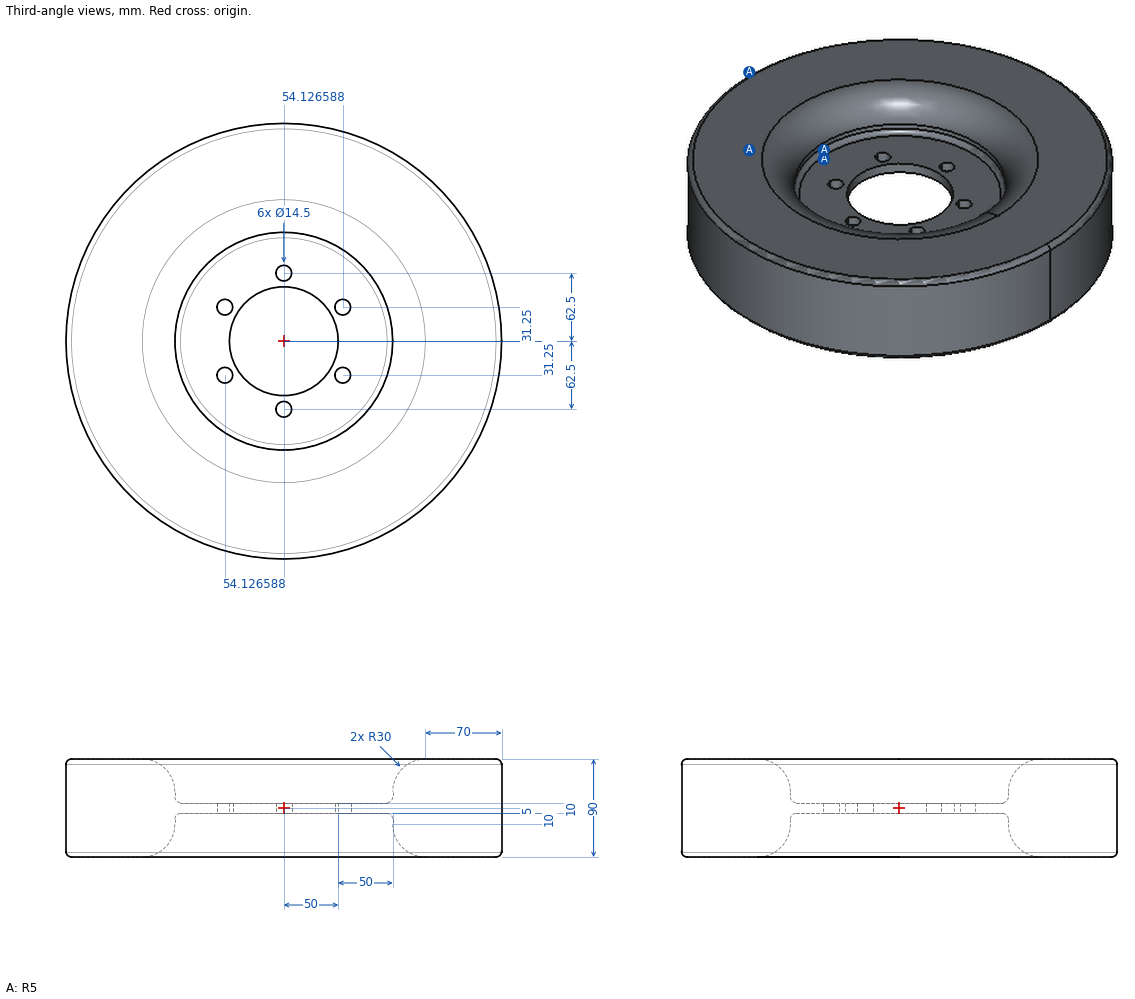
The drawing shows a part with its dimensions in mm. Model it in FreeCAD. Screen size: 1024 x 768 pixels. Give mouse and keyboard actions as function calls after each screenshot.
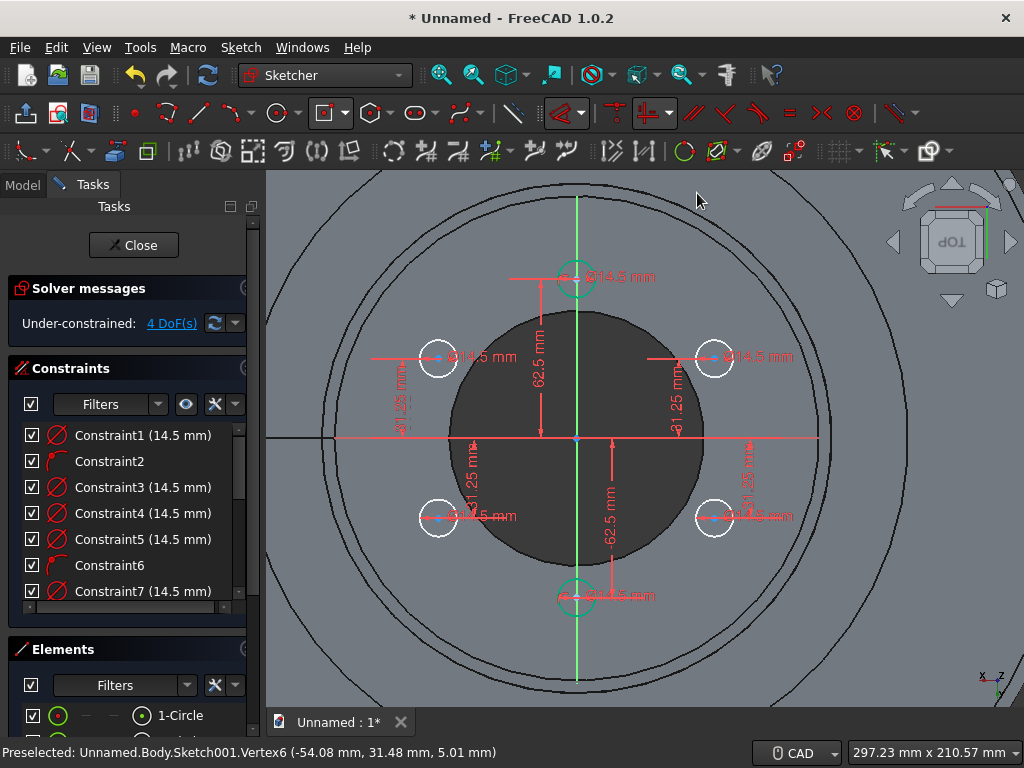
click(438, 518)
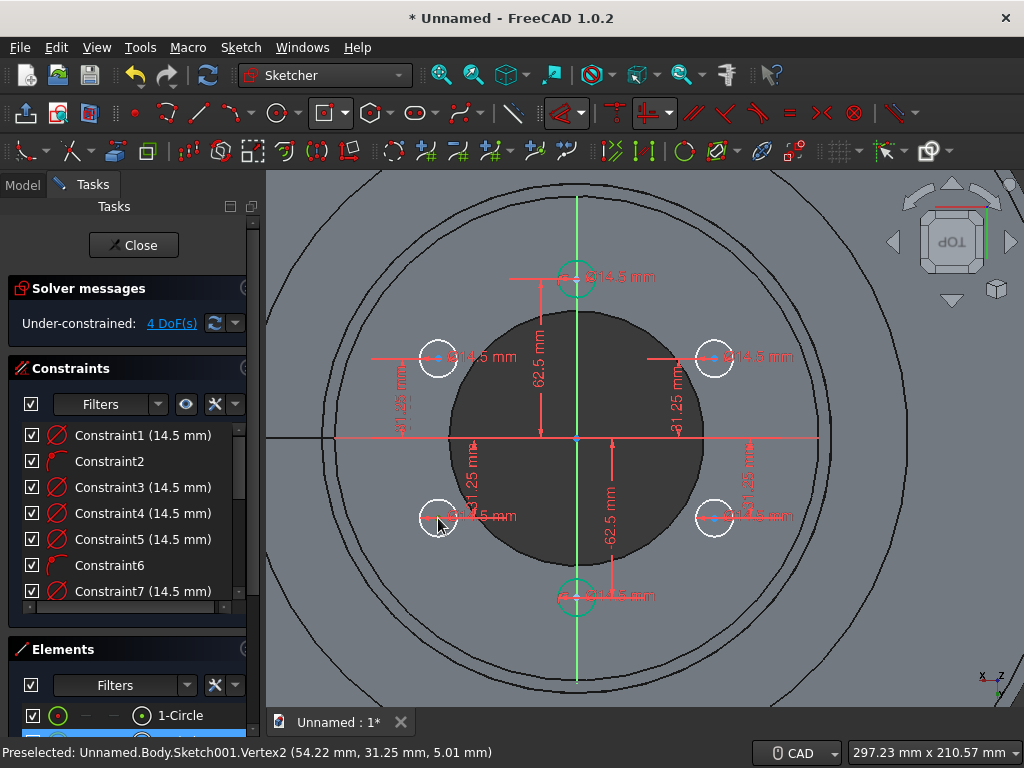
click(584, 114)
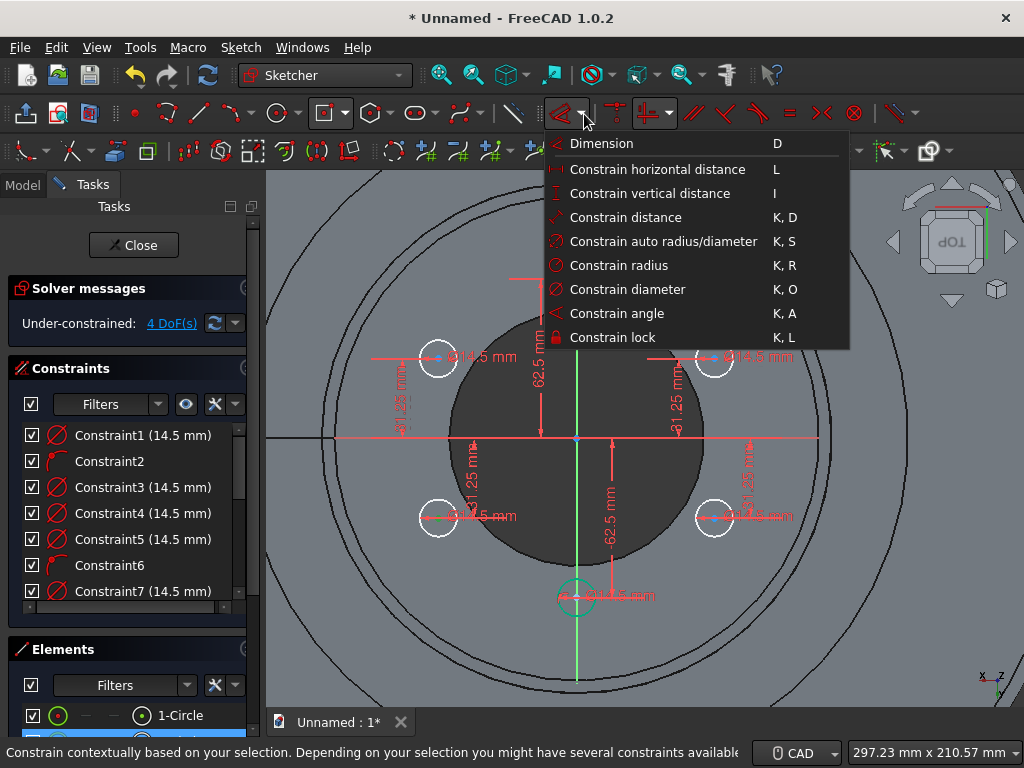
click(697, 169)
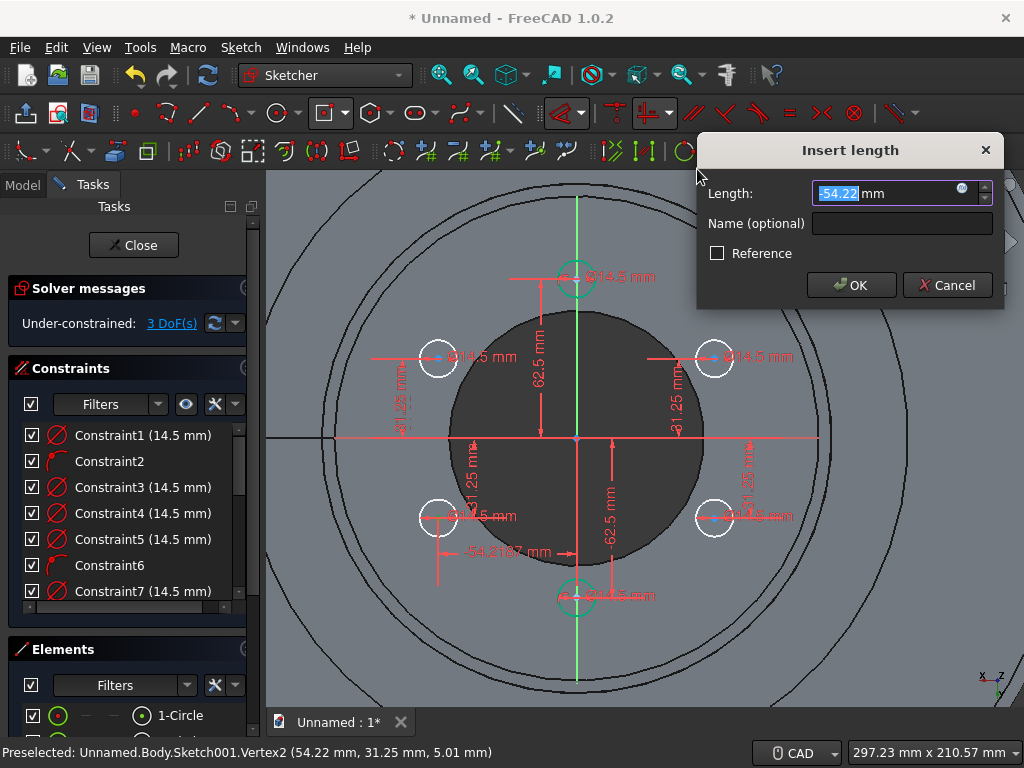
text(-54.126588)
key(Return)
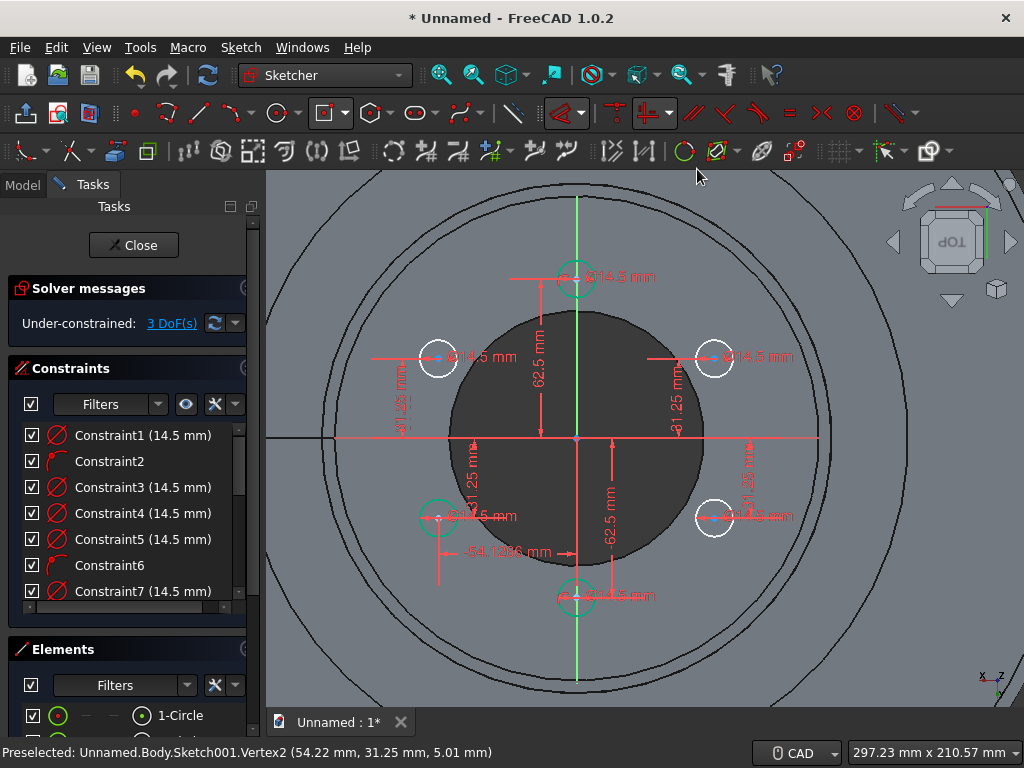
click(438, 359)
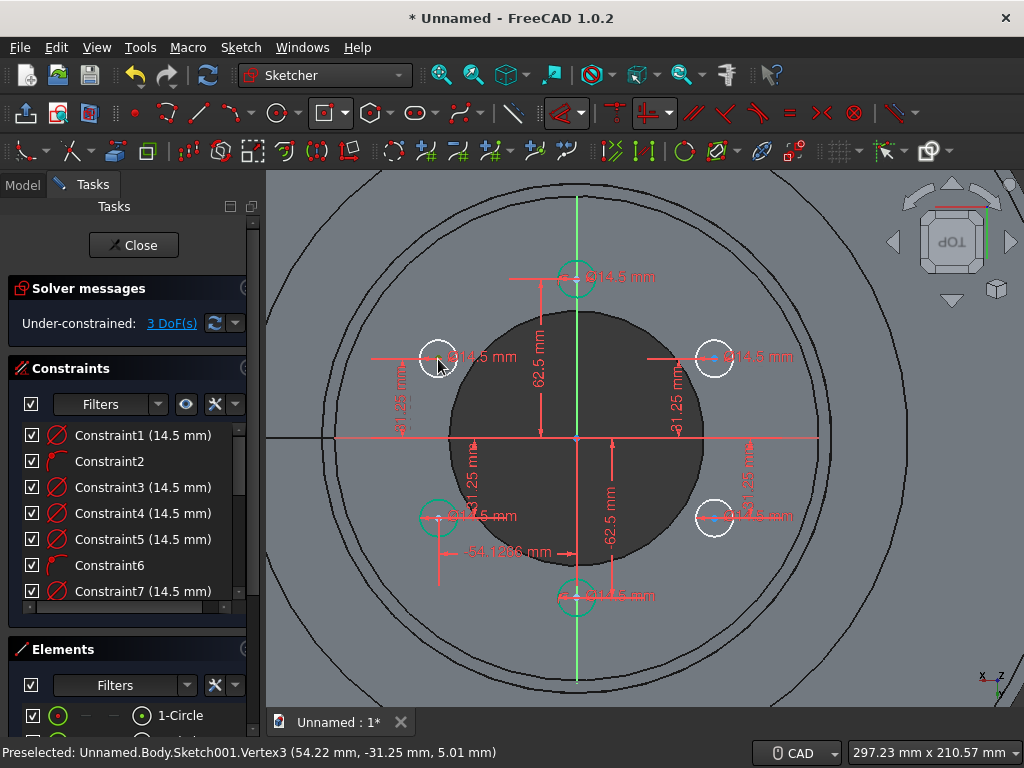
key(l)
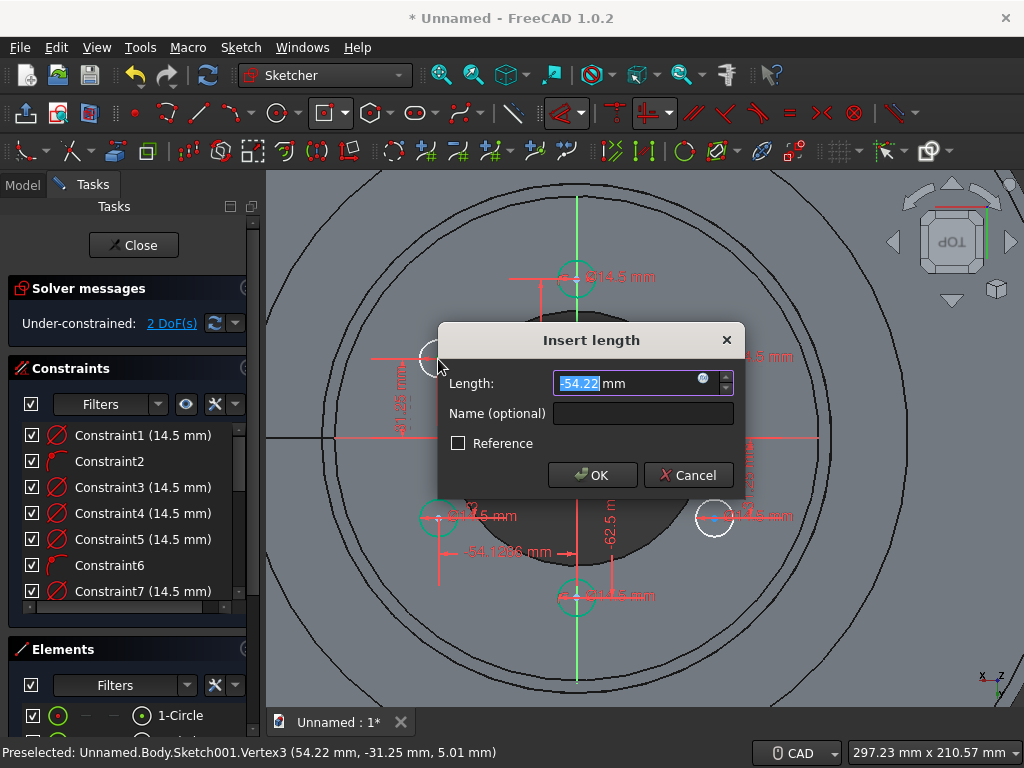
text(-54.126588)
key(Return)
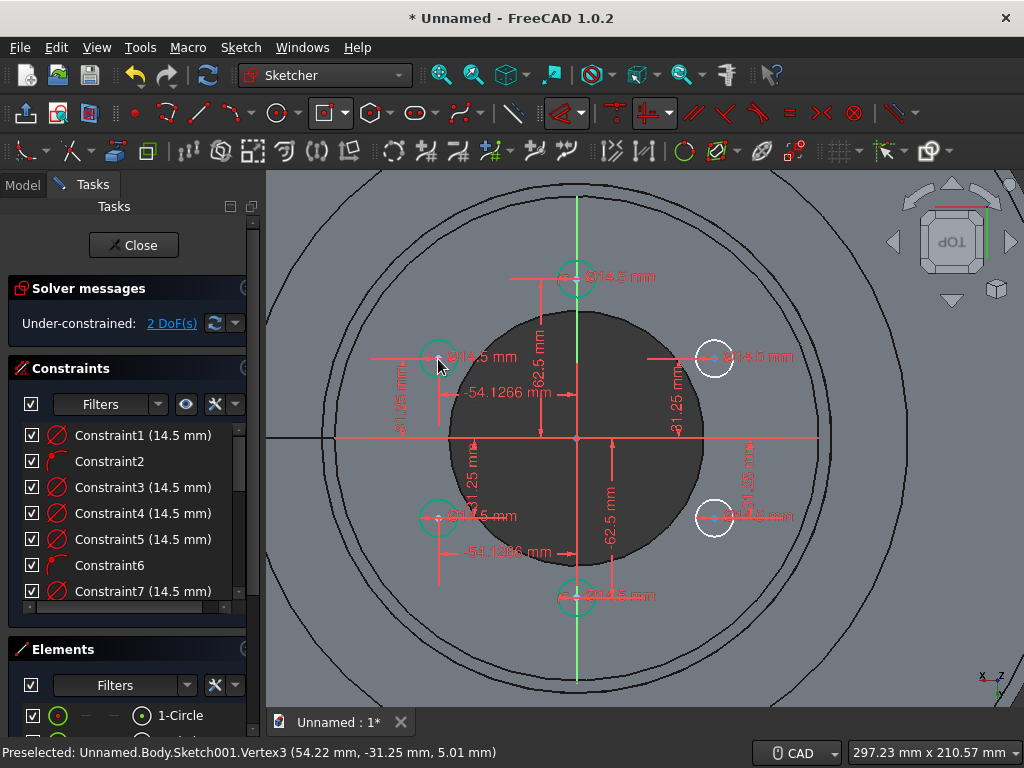
click(715, 359)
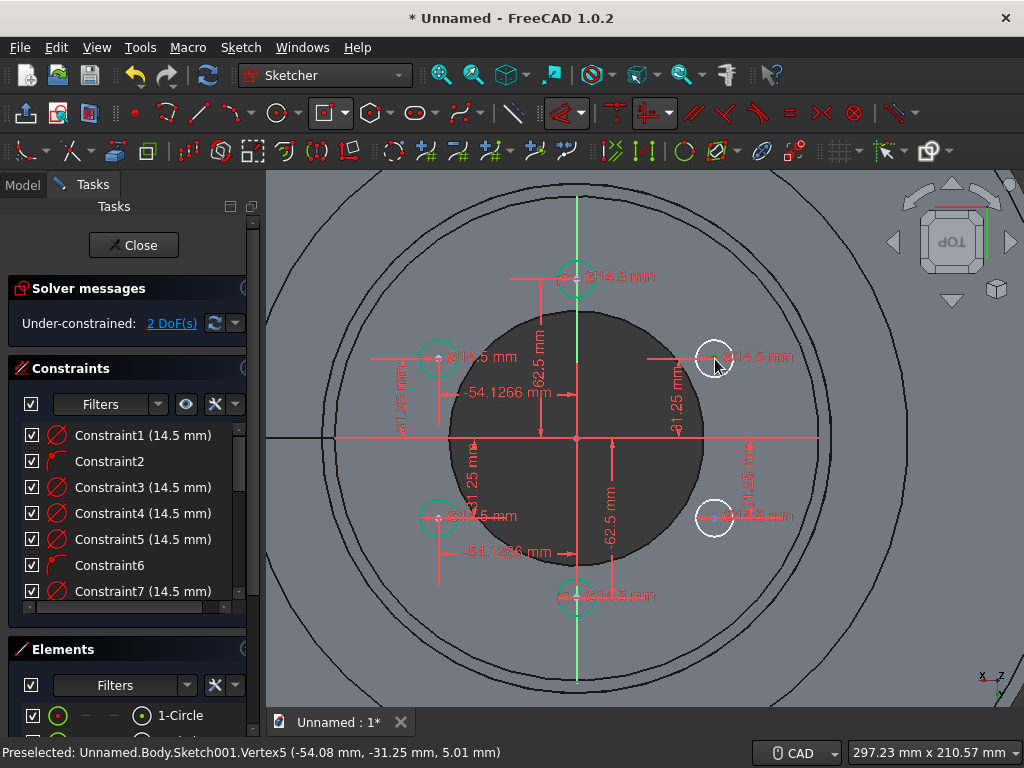
click(584, 114)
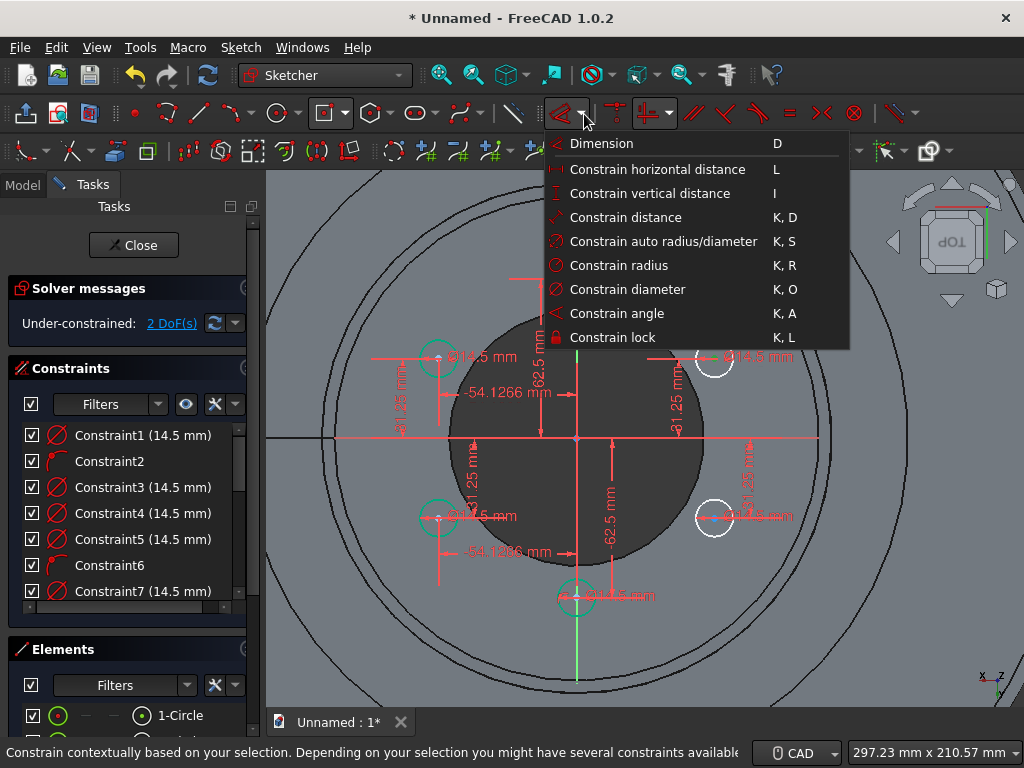
click(697, 169)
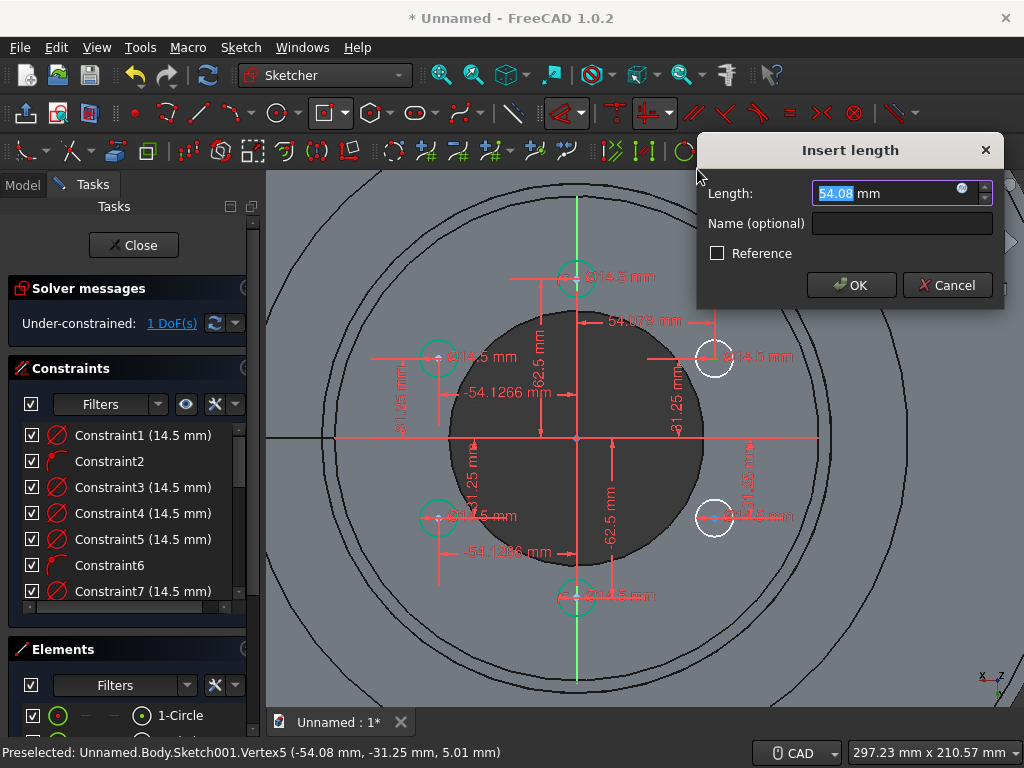
text(54.126588)
key(Return)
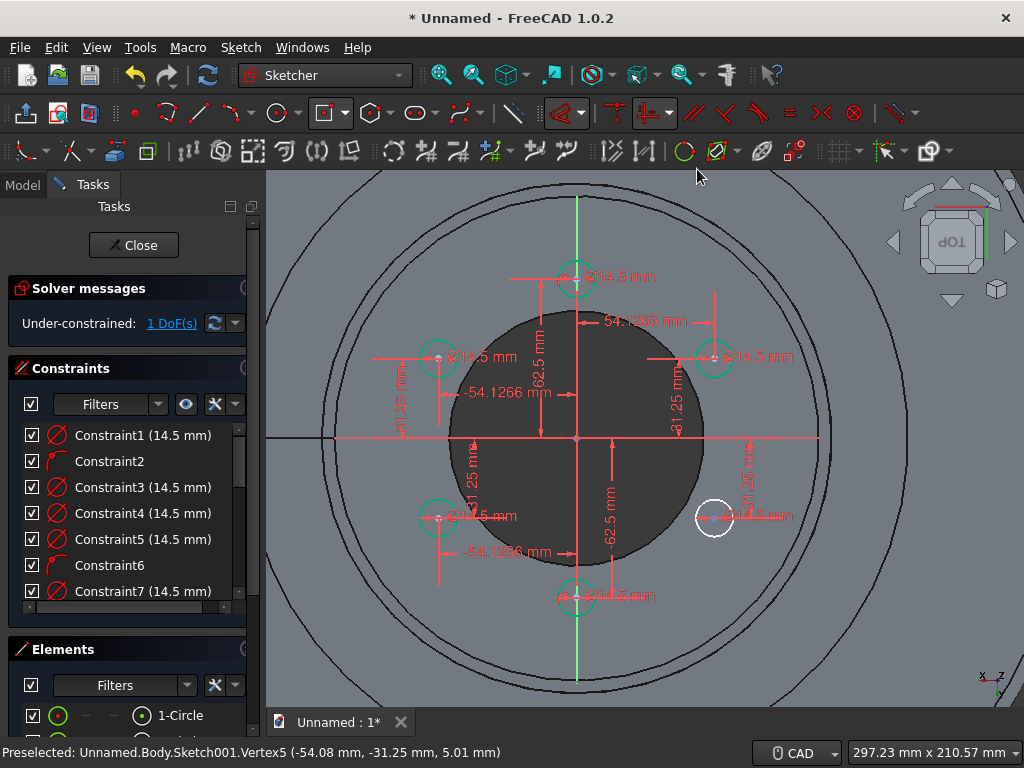
click(715, 518)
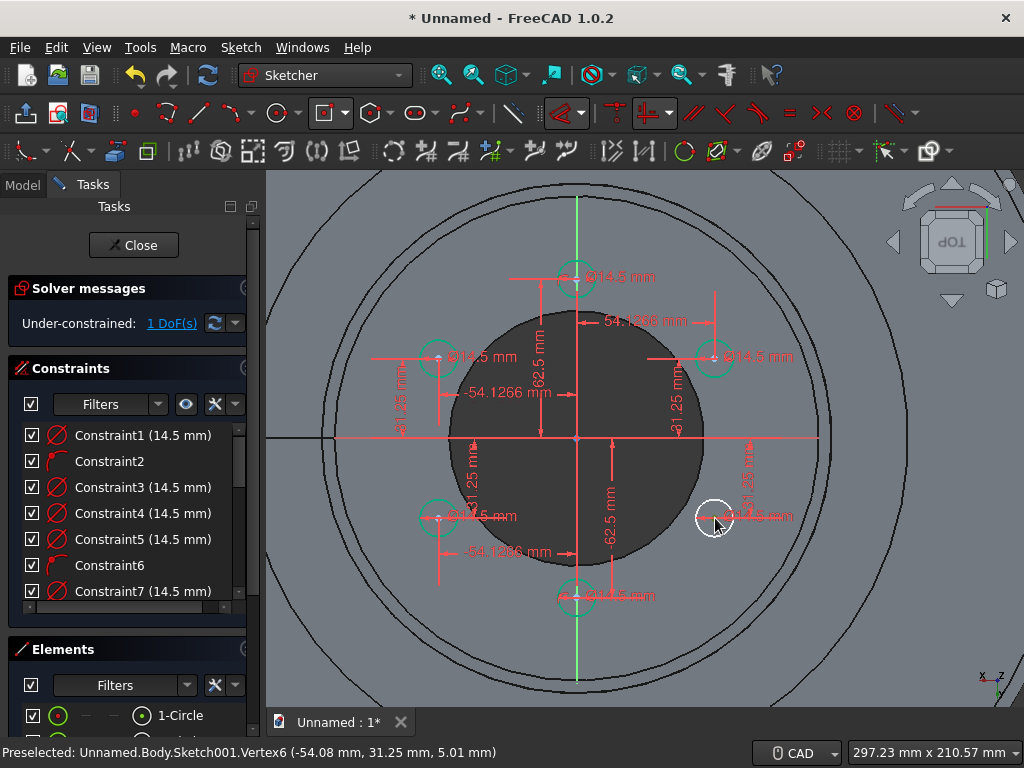
key(l)